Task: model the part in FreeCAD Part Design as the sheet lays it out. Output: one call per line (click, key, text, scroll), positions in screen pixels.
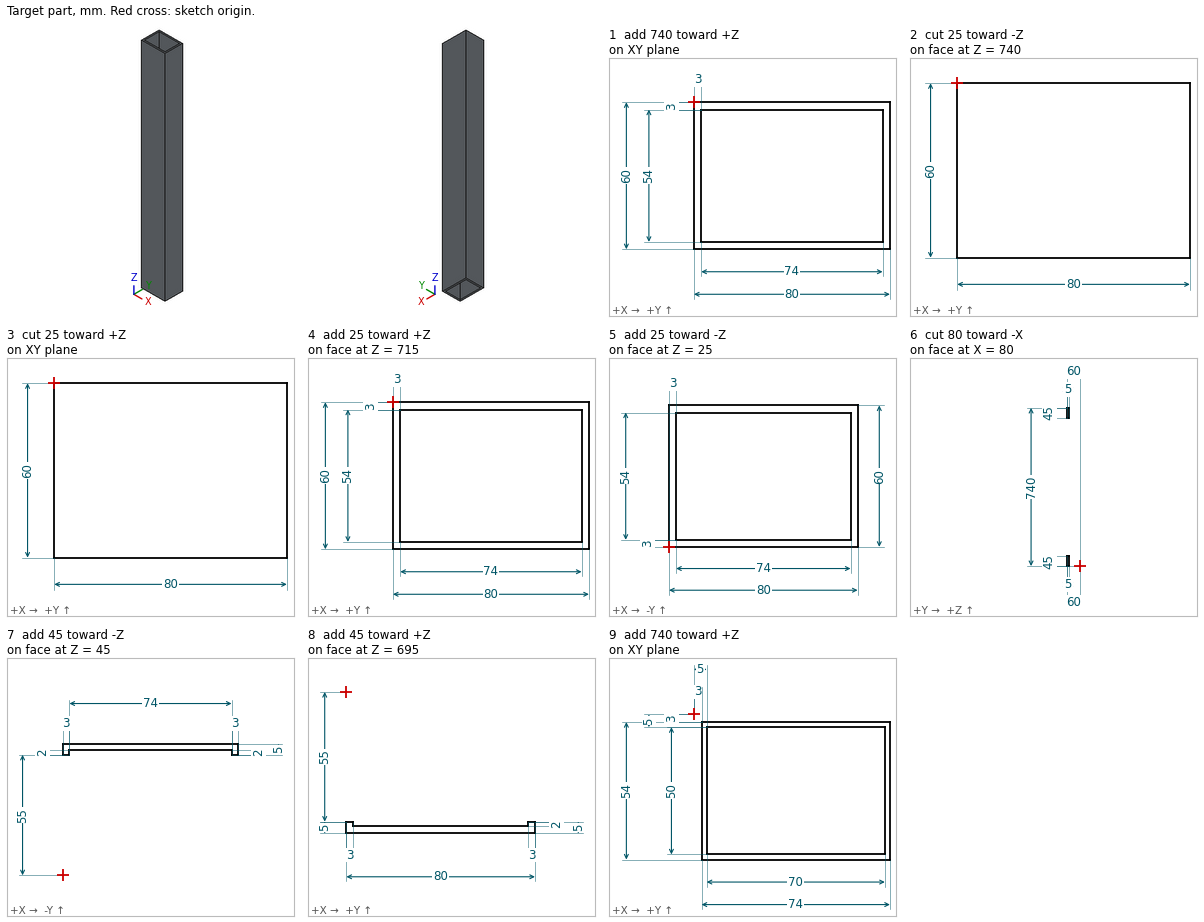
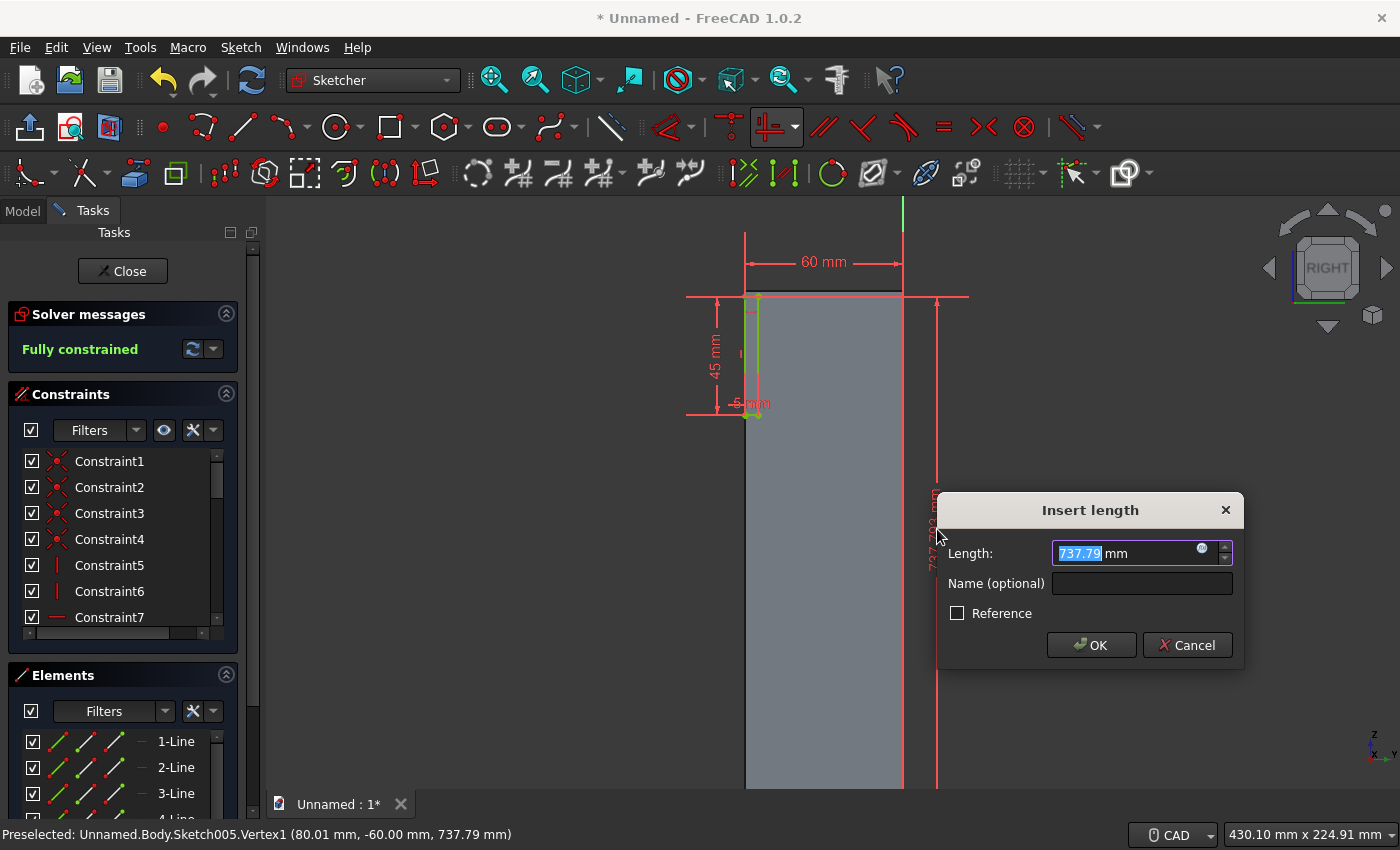
text(740)
key(Return)
key(Escape)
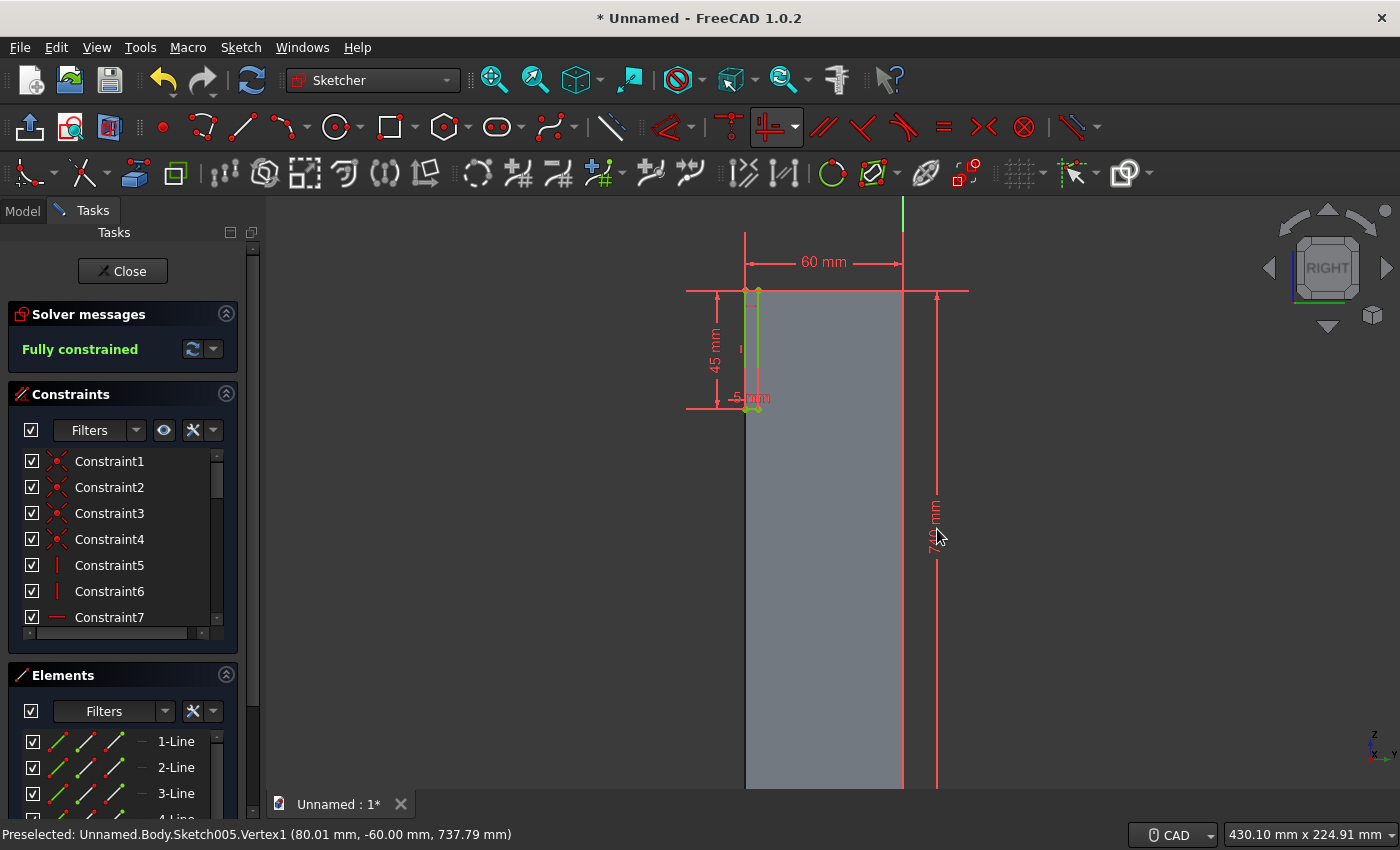
click(123, 271)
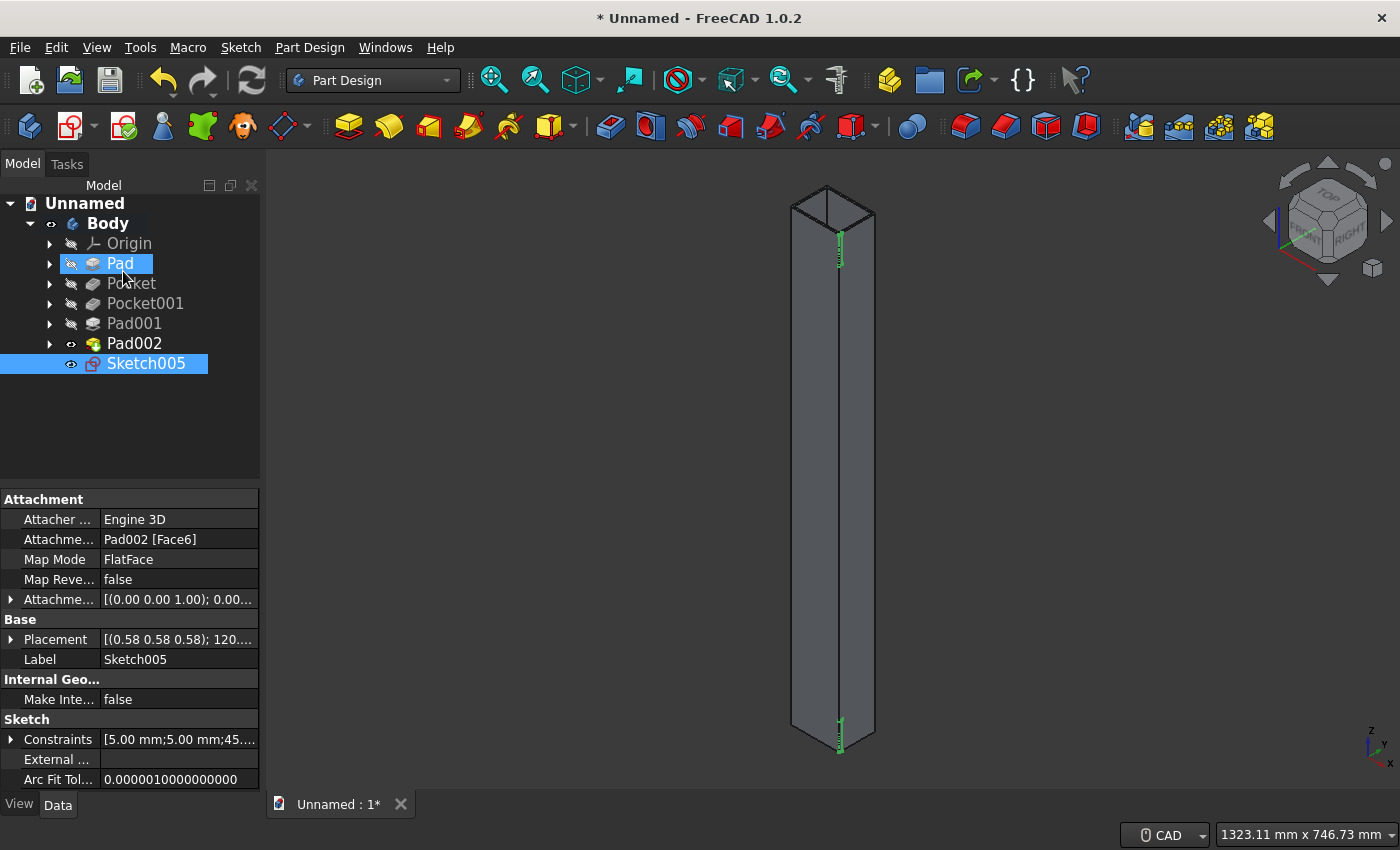
click(612, 126)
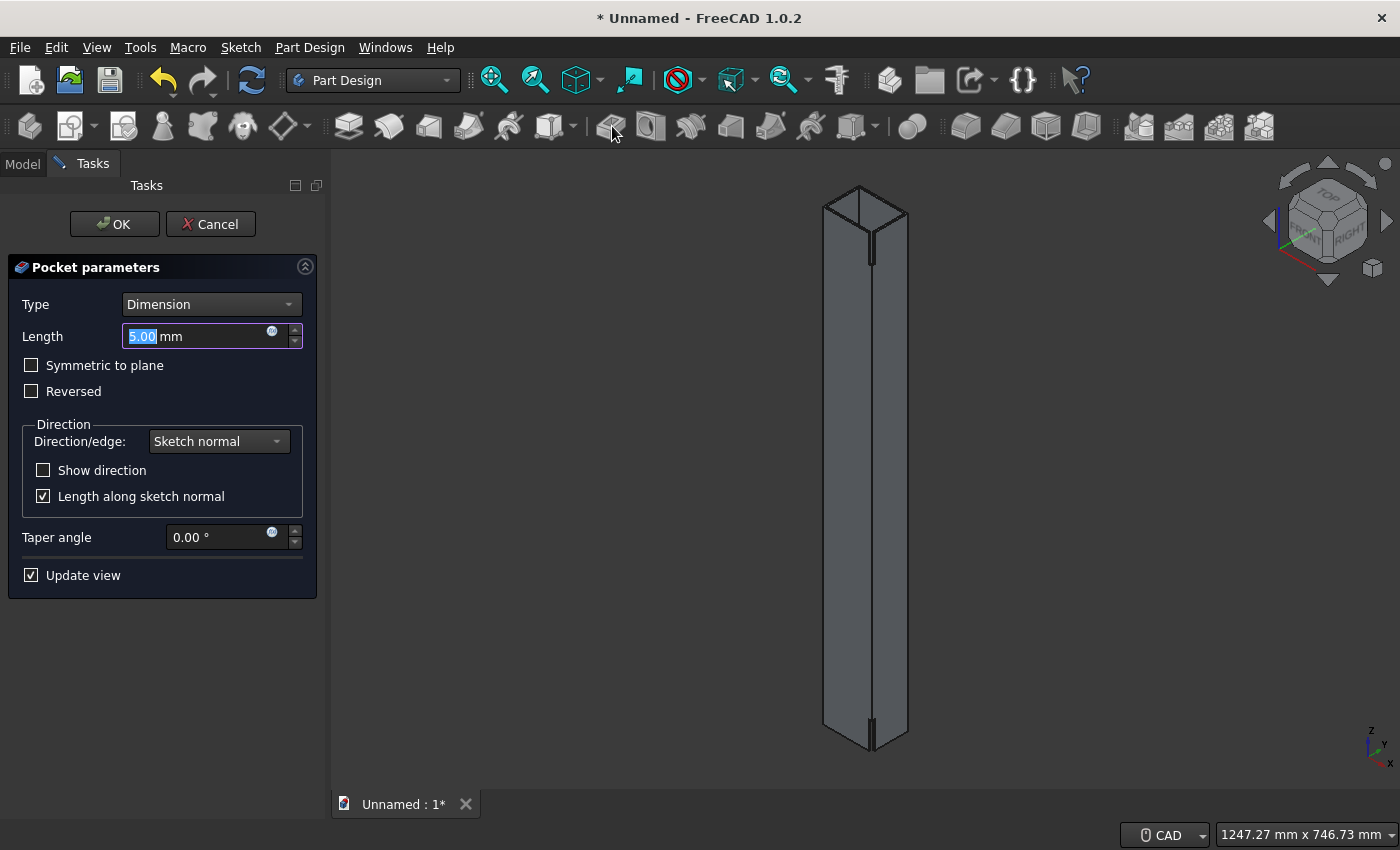
text(80)
key(Tab)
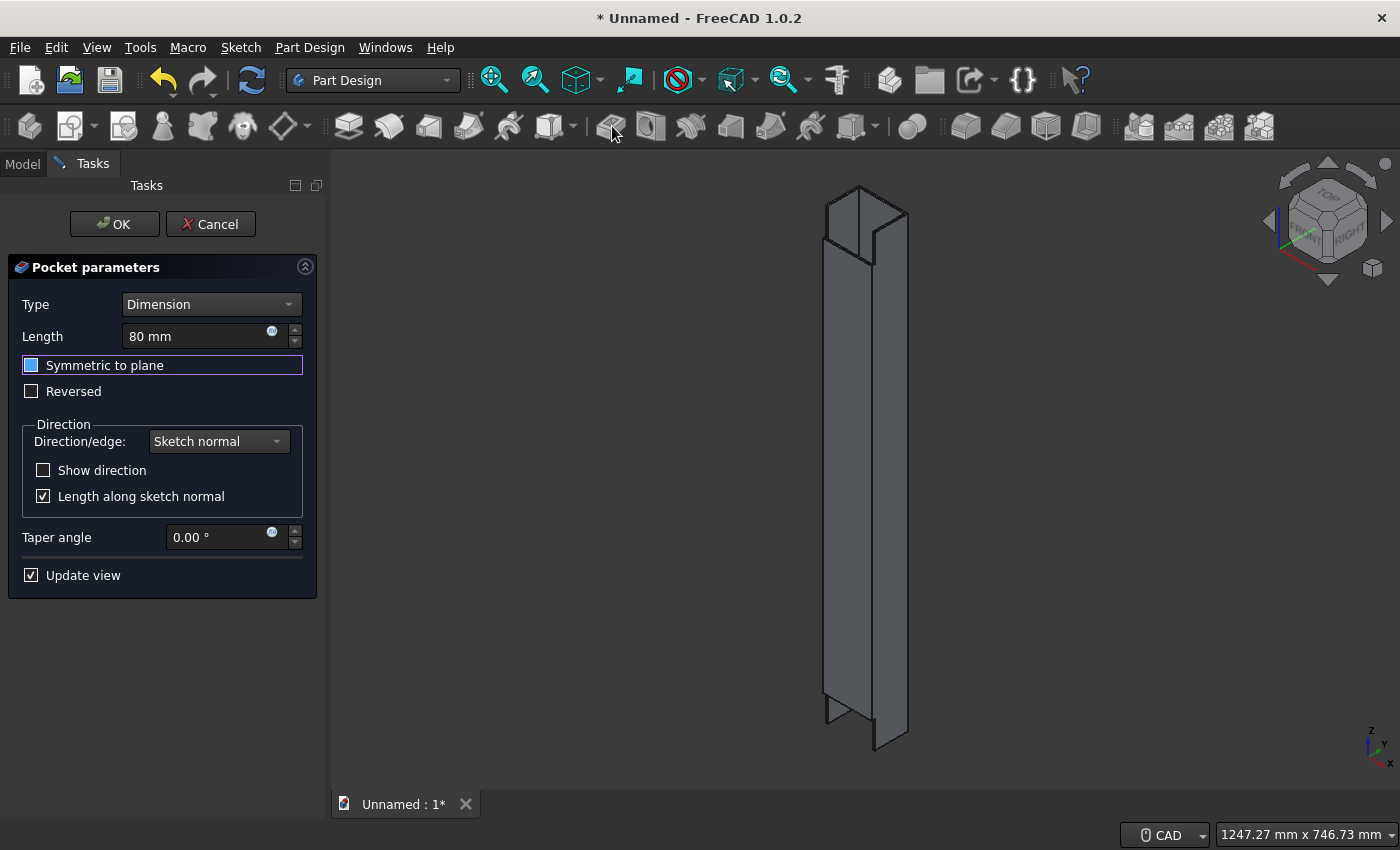
click(115, 224)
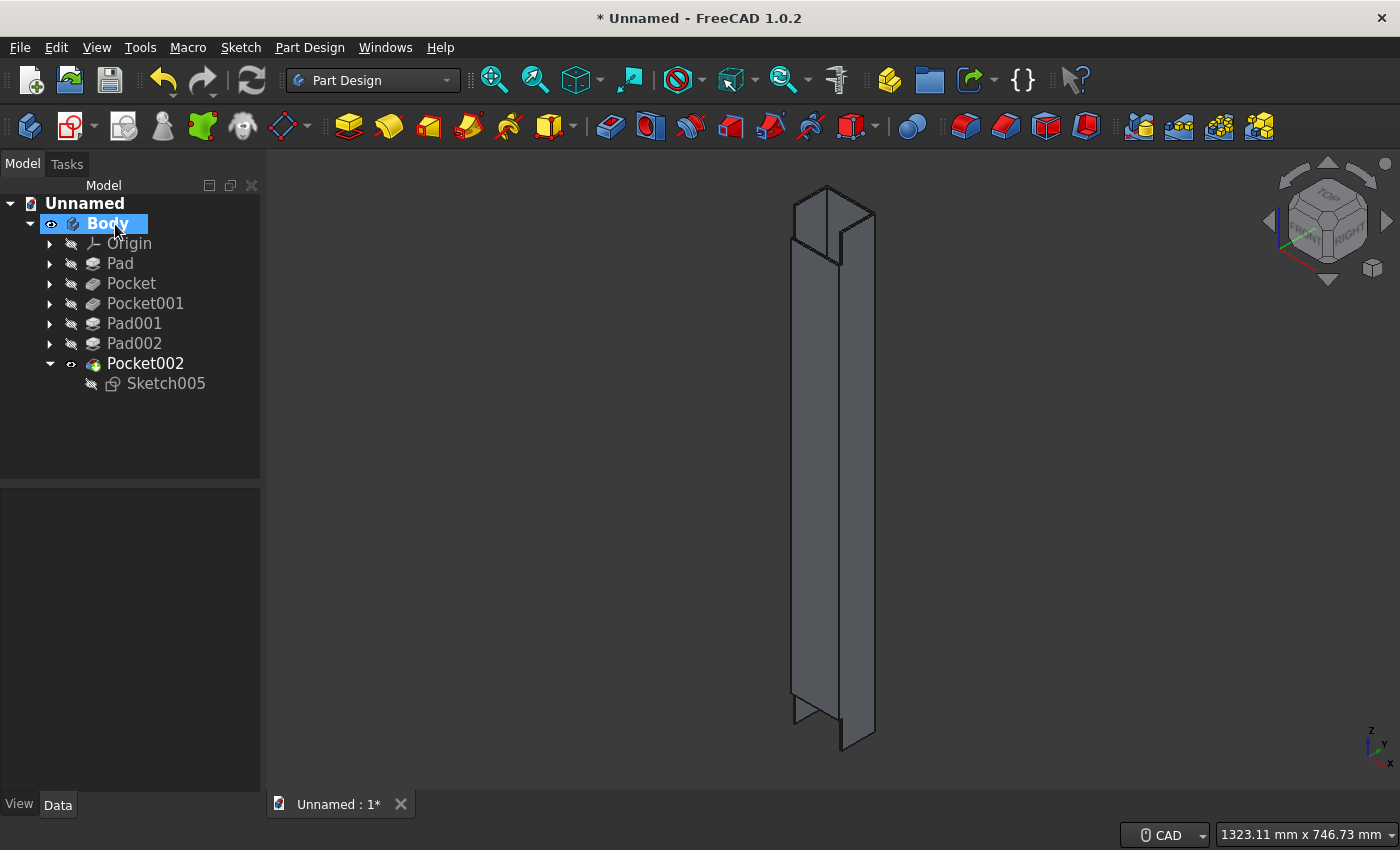
key(5)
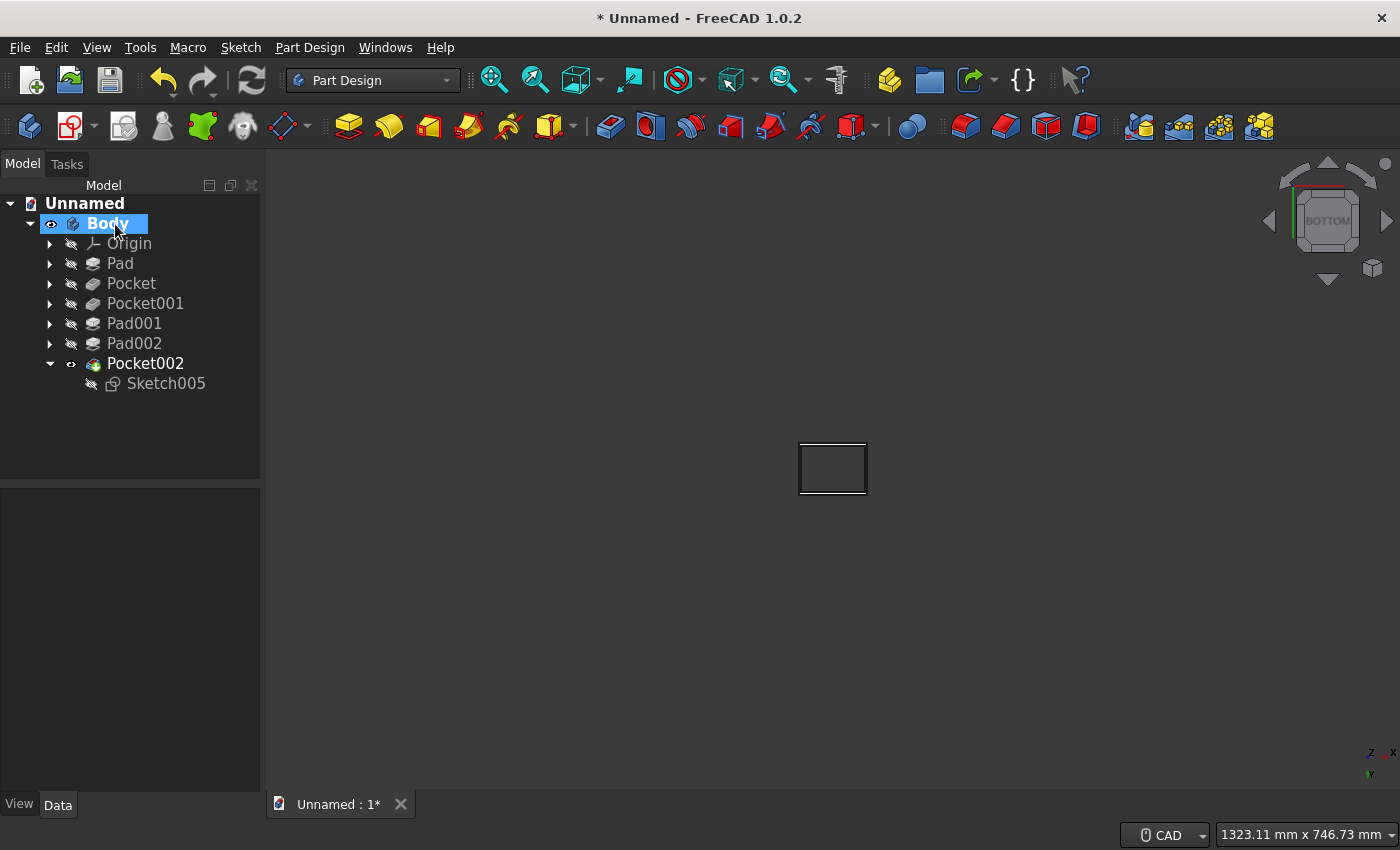
key(v)
key(f)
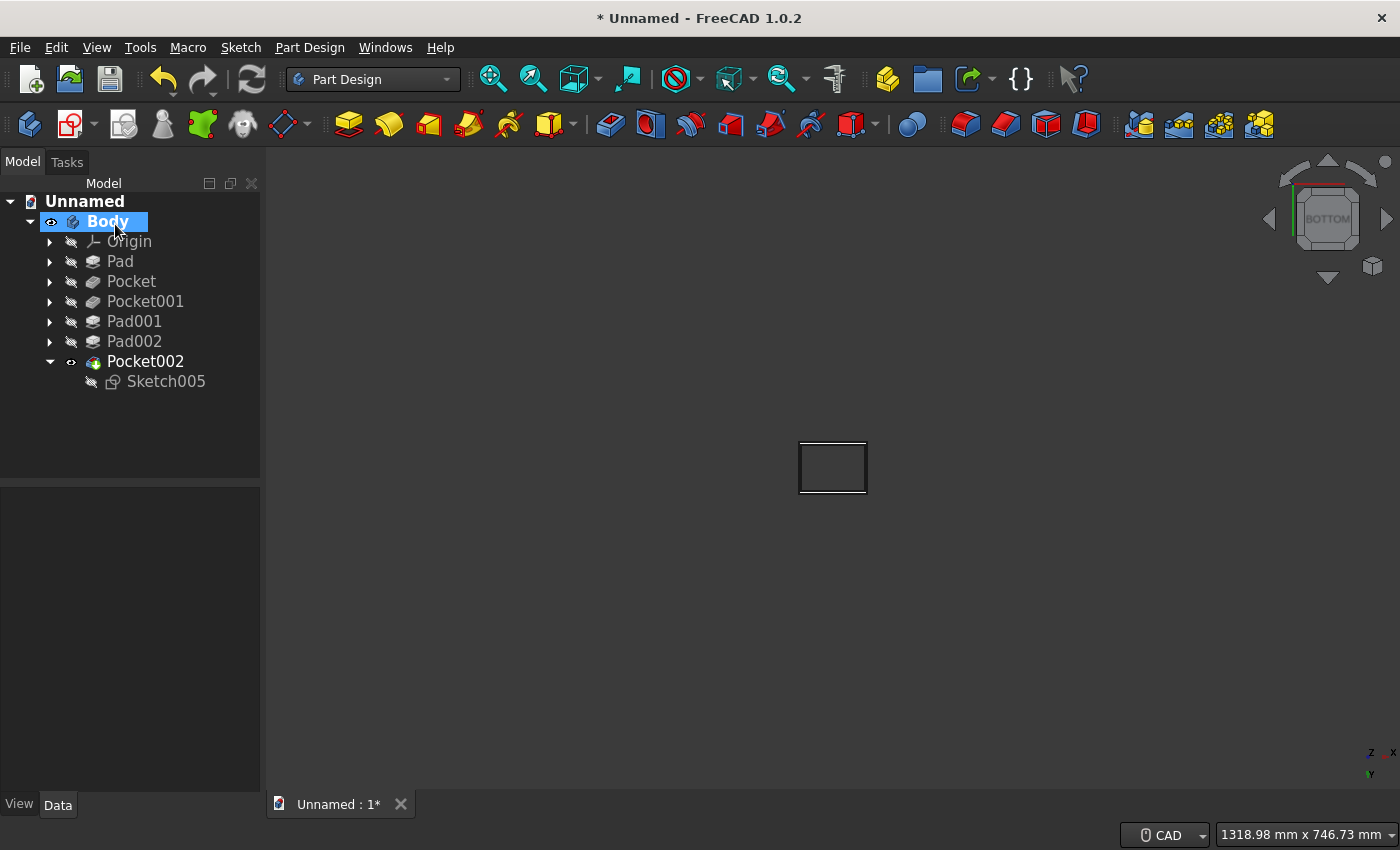
scroll(862, 443, up, 13)